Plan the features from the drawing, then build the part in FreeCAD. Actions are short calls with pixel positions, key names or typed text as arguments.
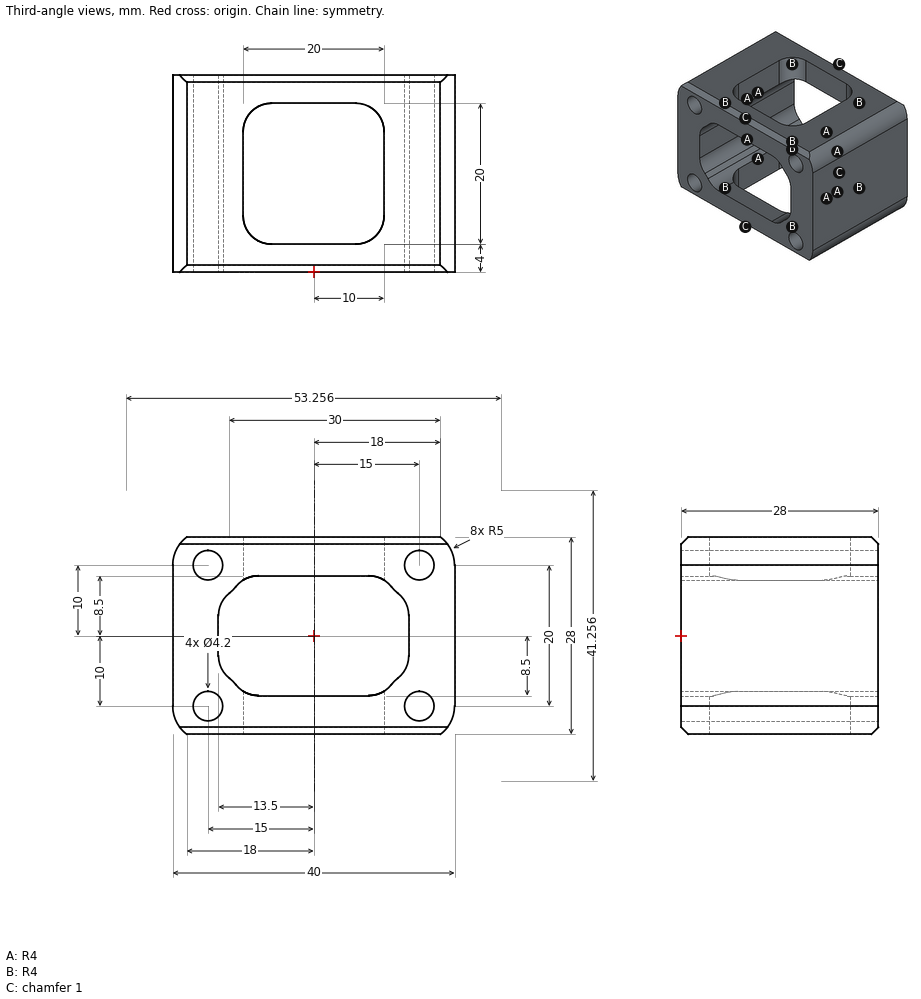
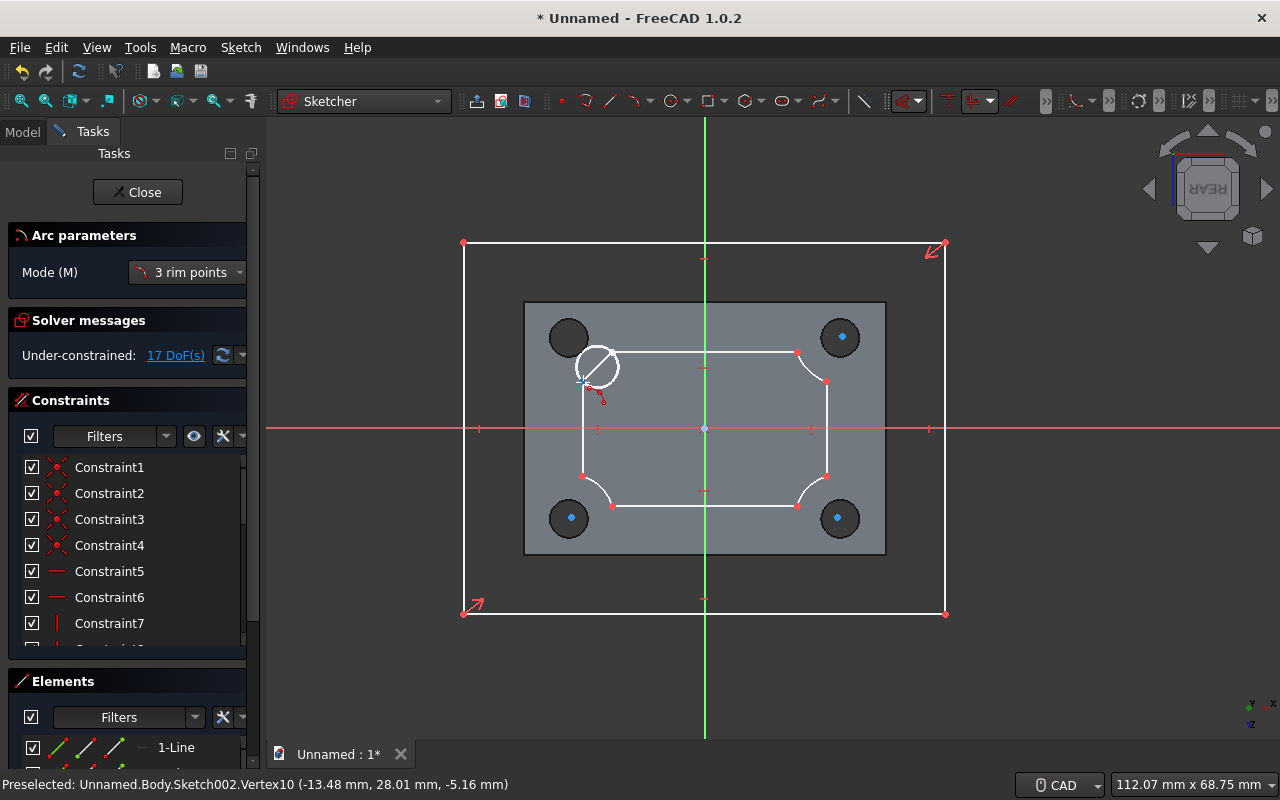
scroll(601, 370, up, 6)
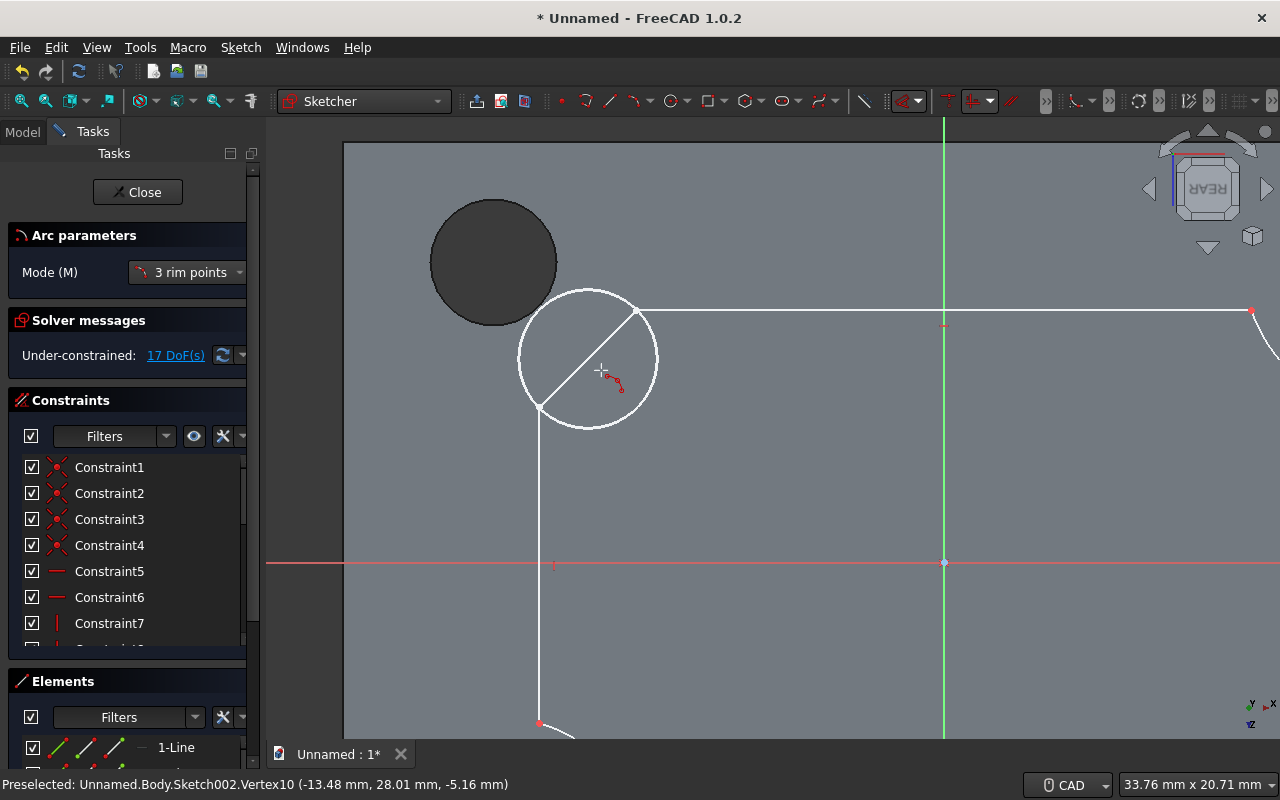
click(600, 369)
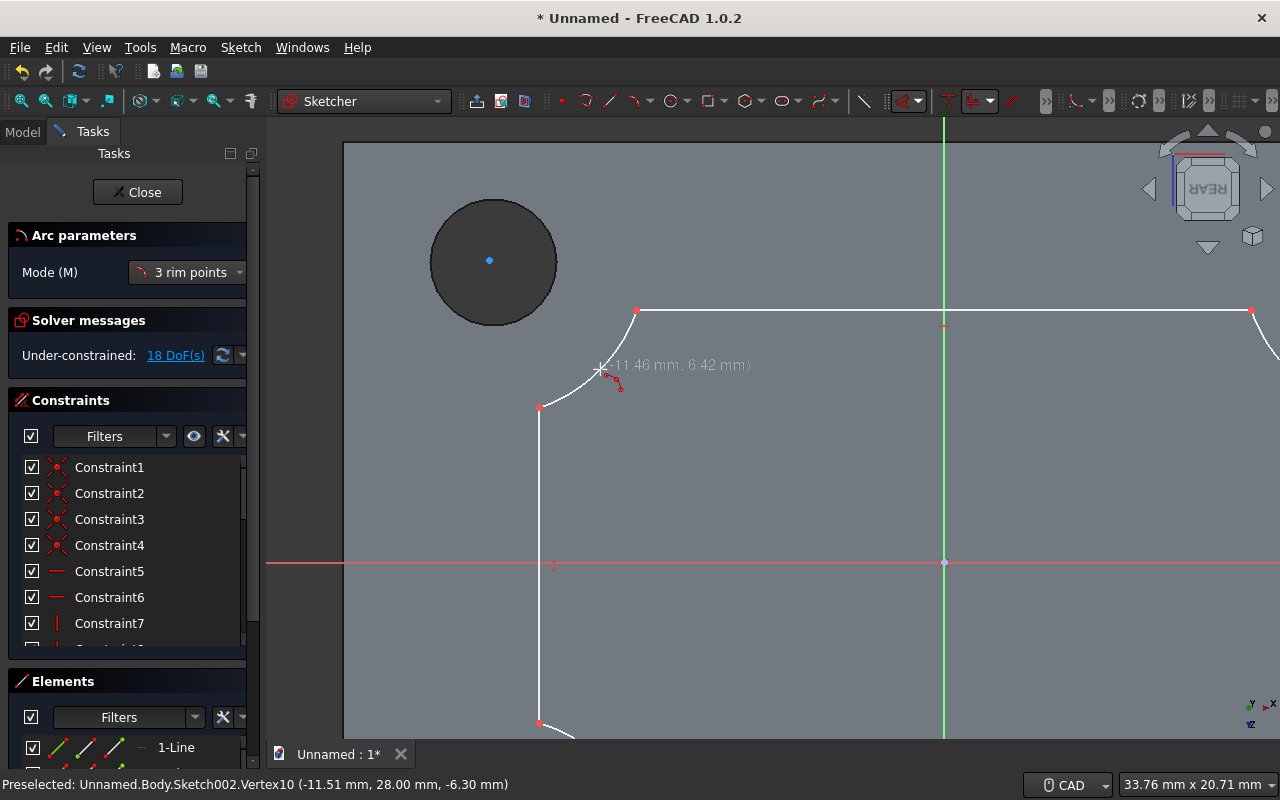
key(g)
key(l)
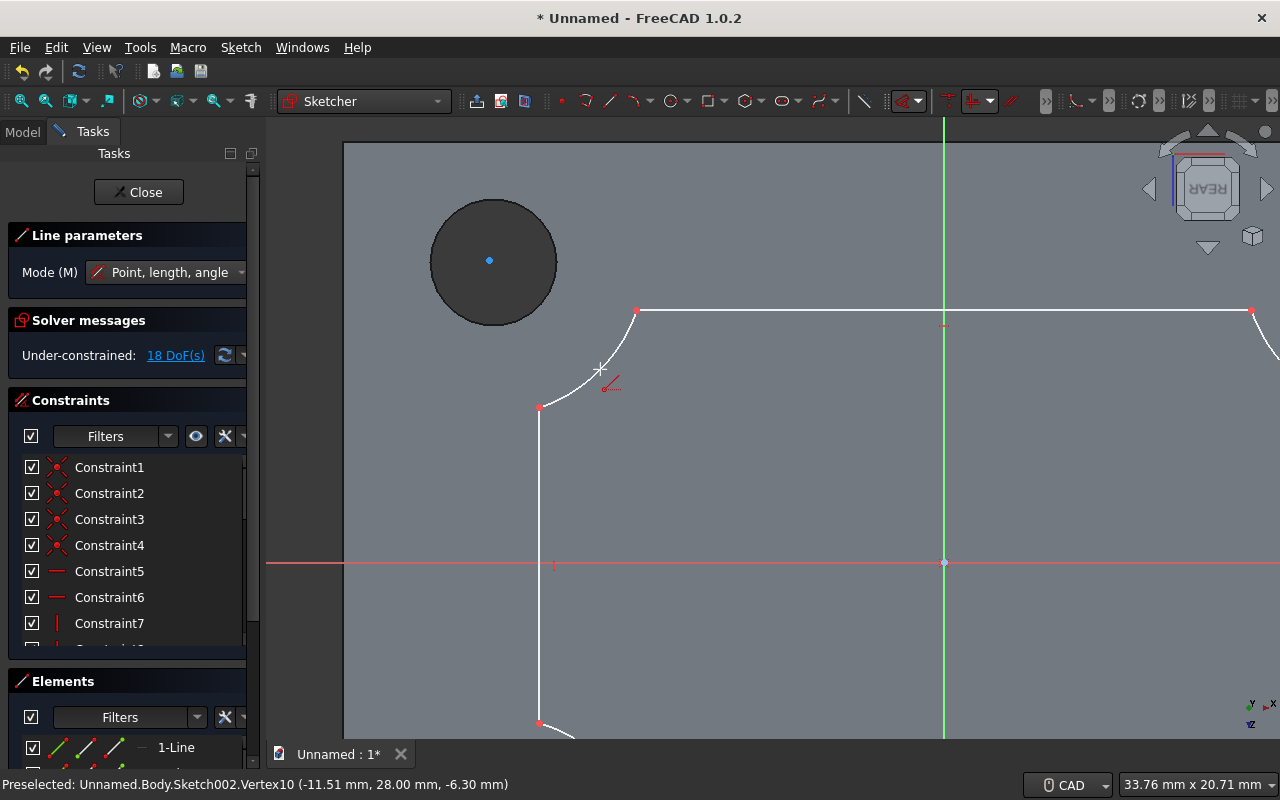
scroll(601, 370, down, 6)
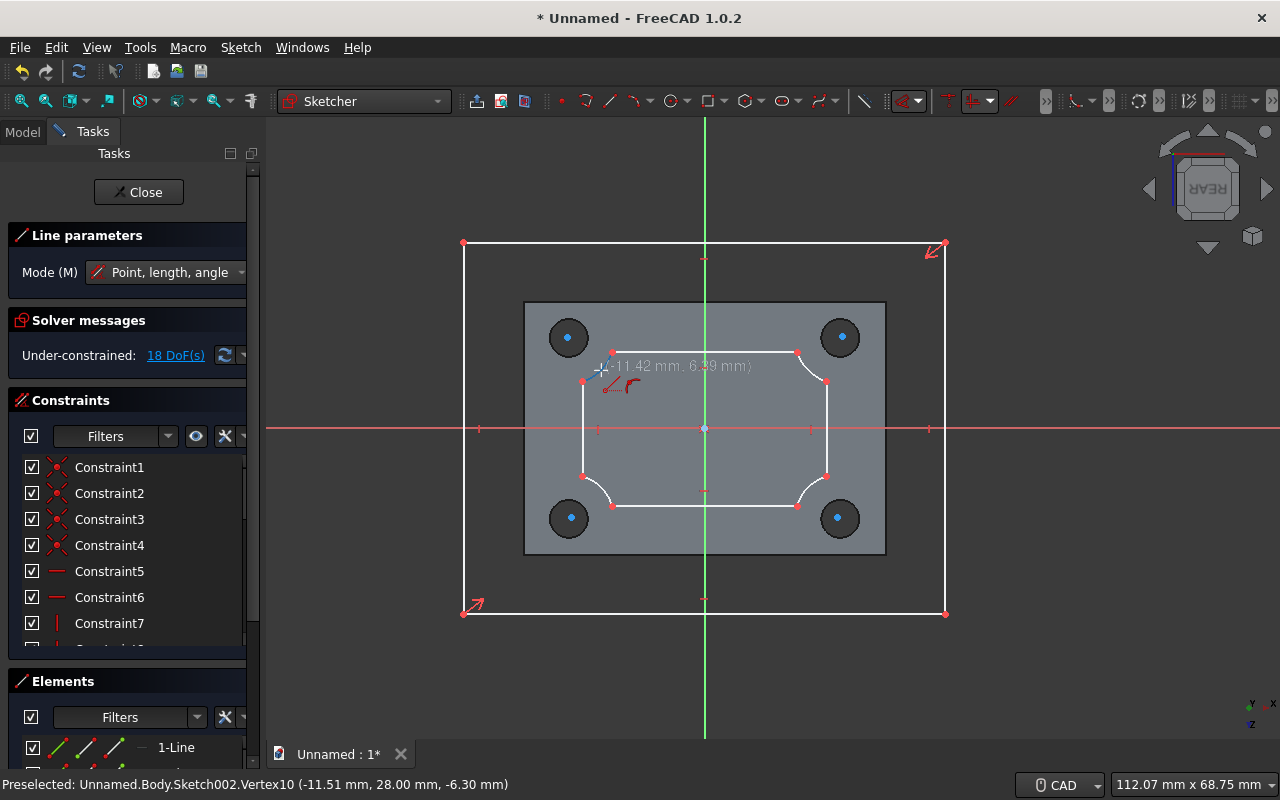
click(886, 338)
click(886, 519)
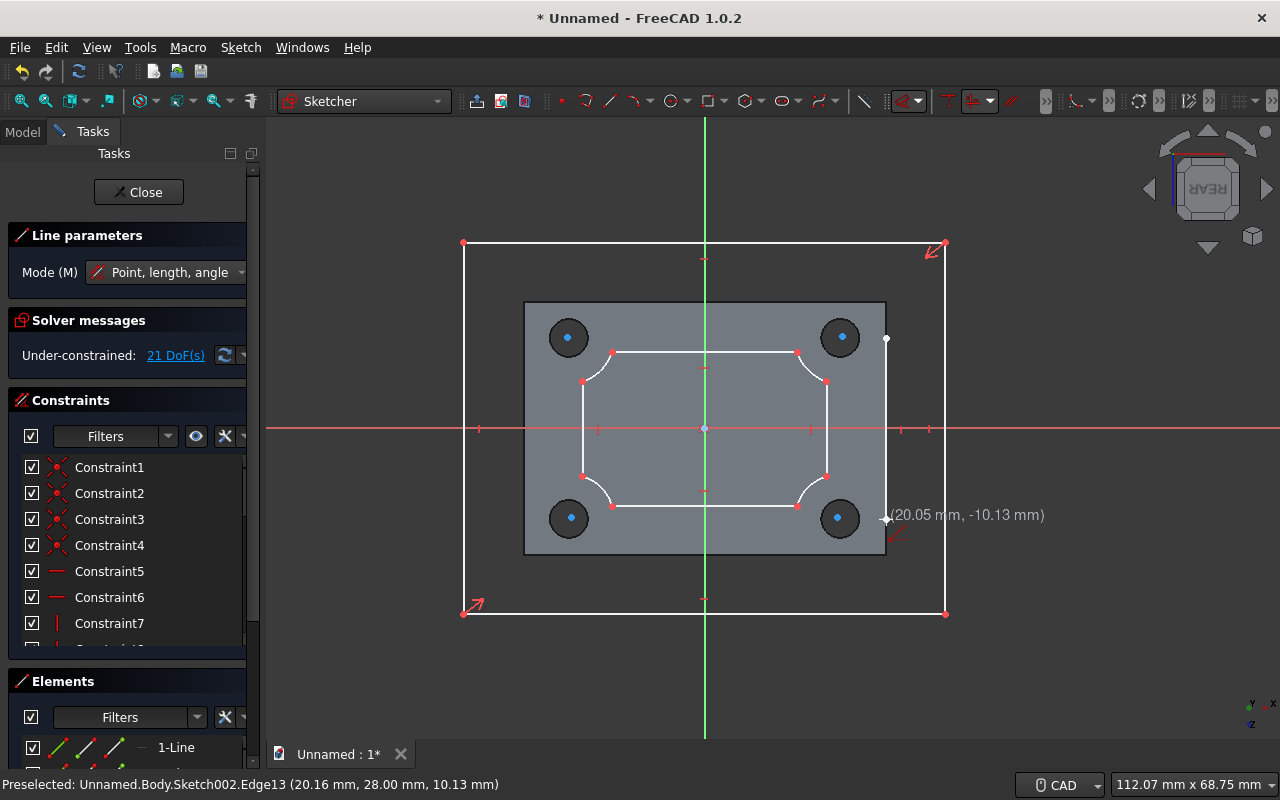
click(867, 555)
click(596, 555)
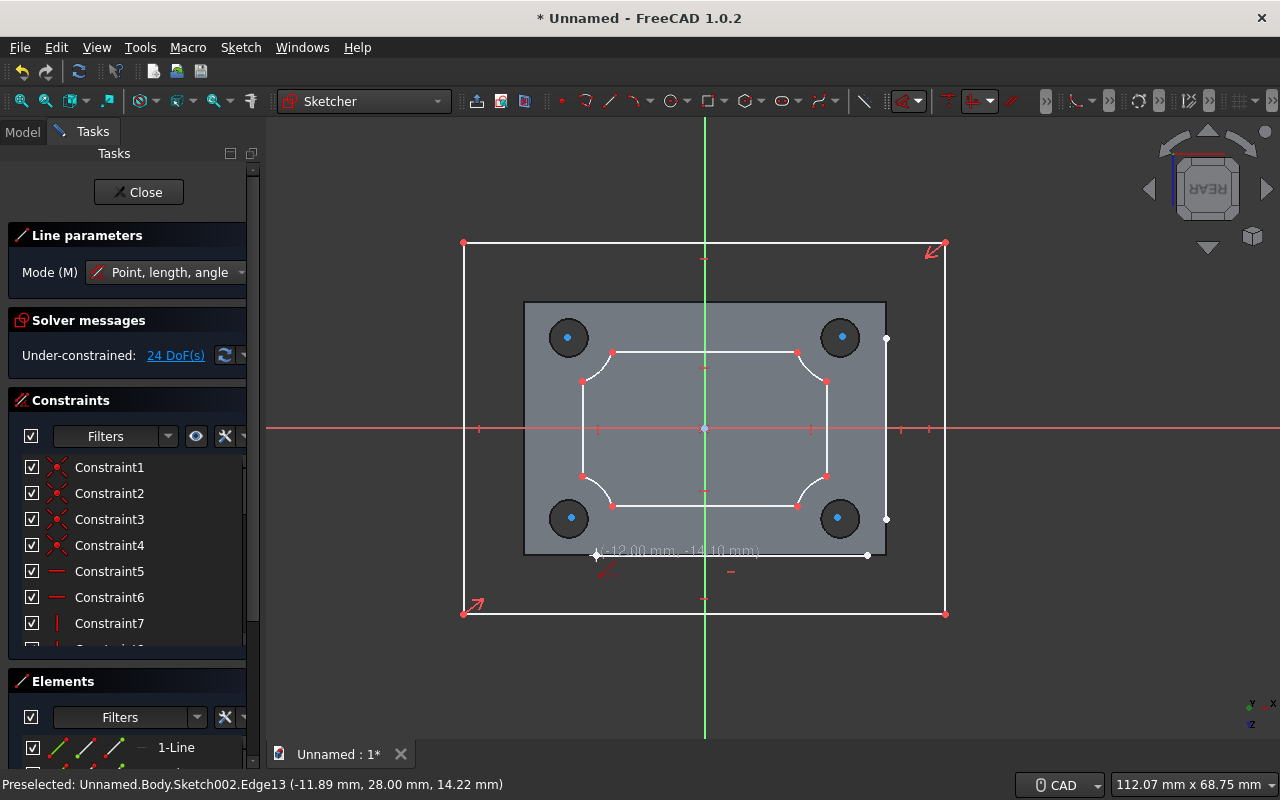
click(524, 519)
click(524, 338)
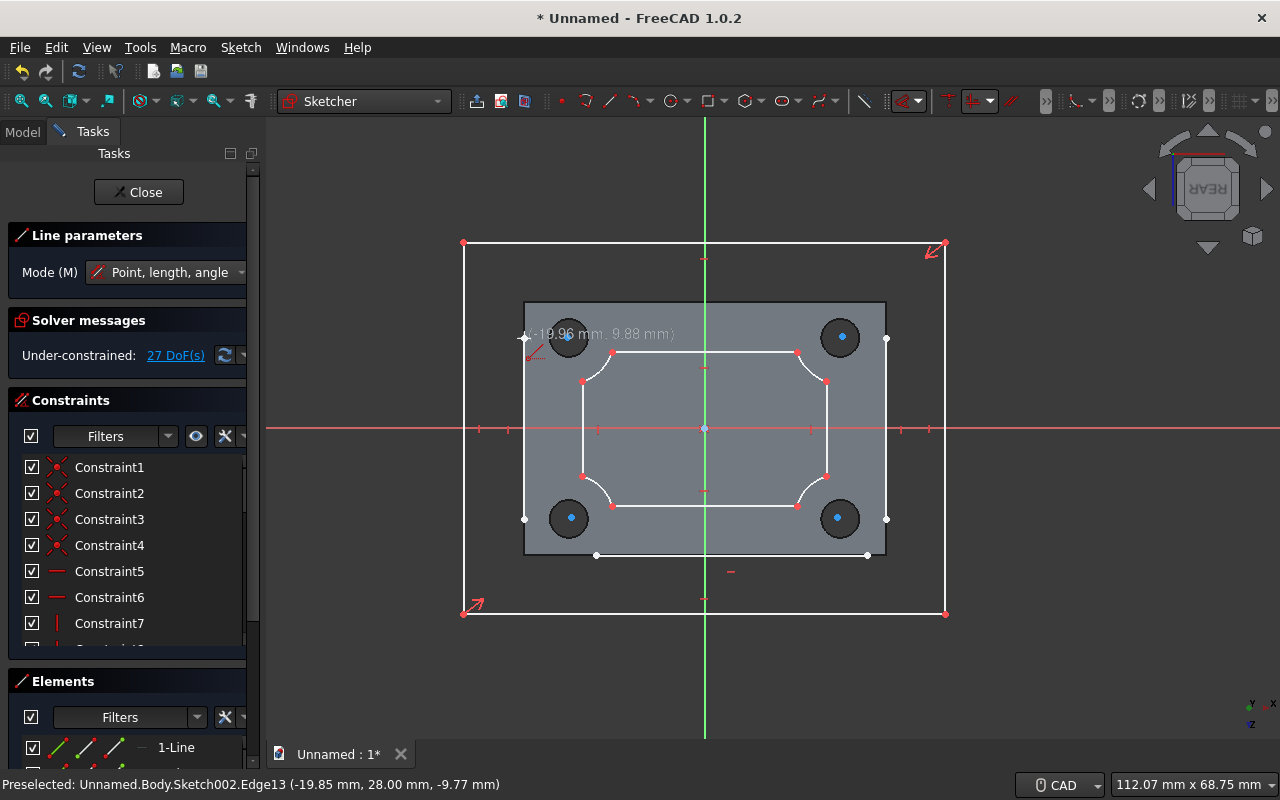
click(542, 302)
click(813, 302)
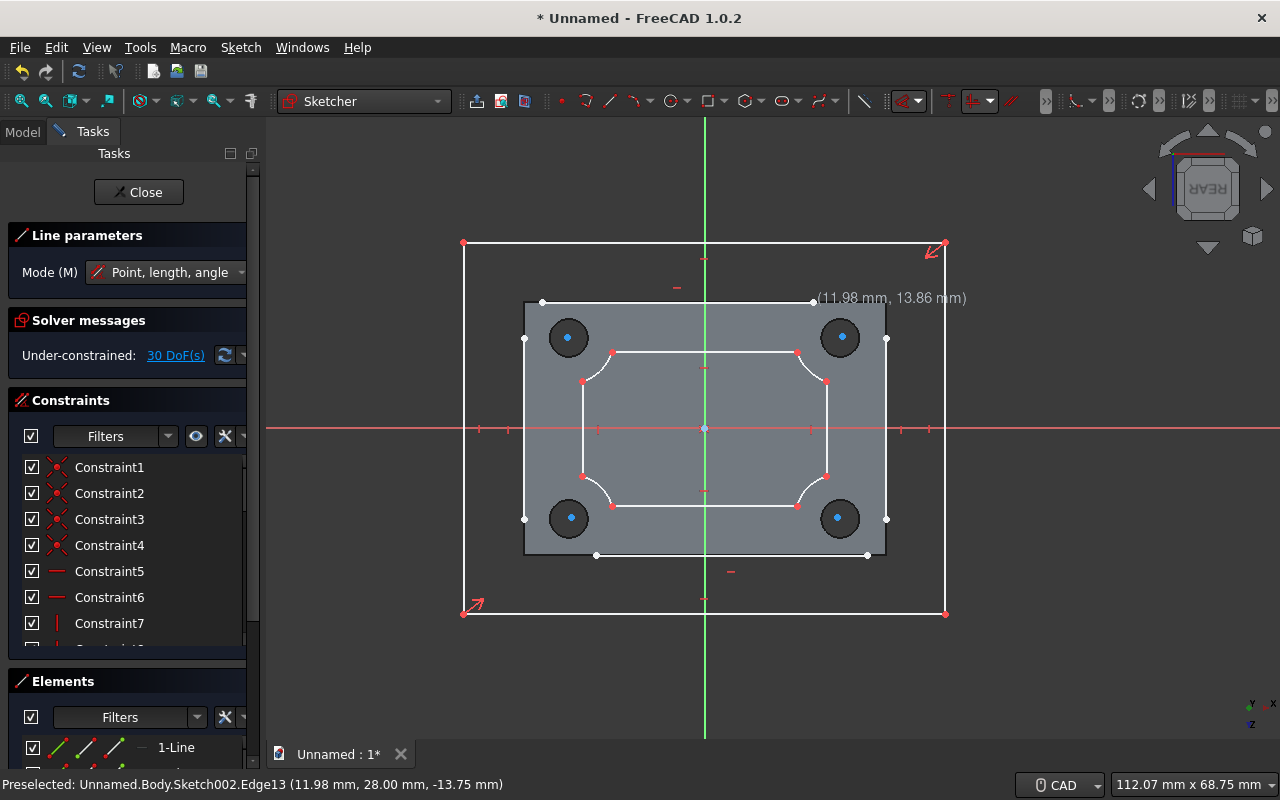
key(g)
key(3)
key(a)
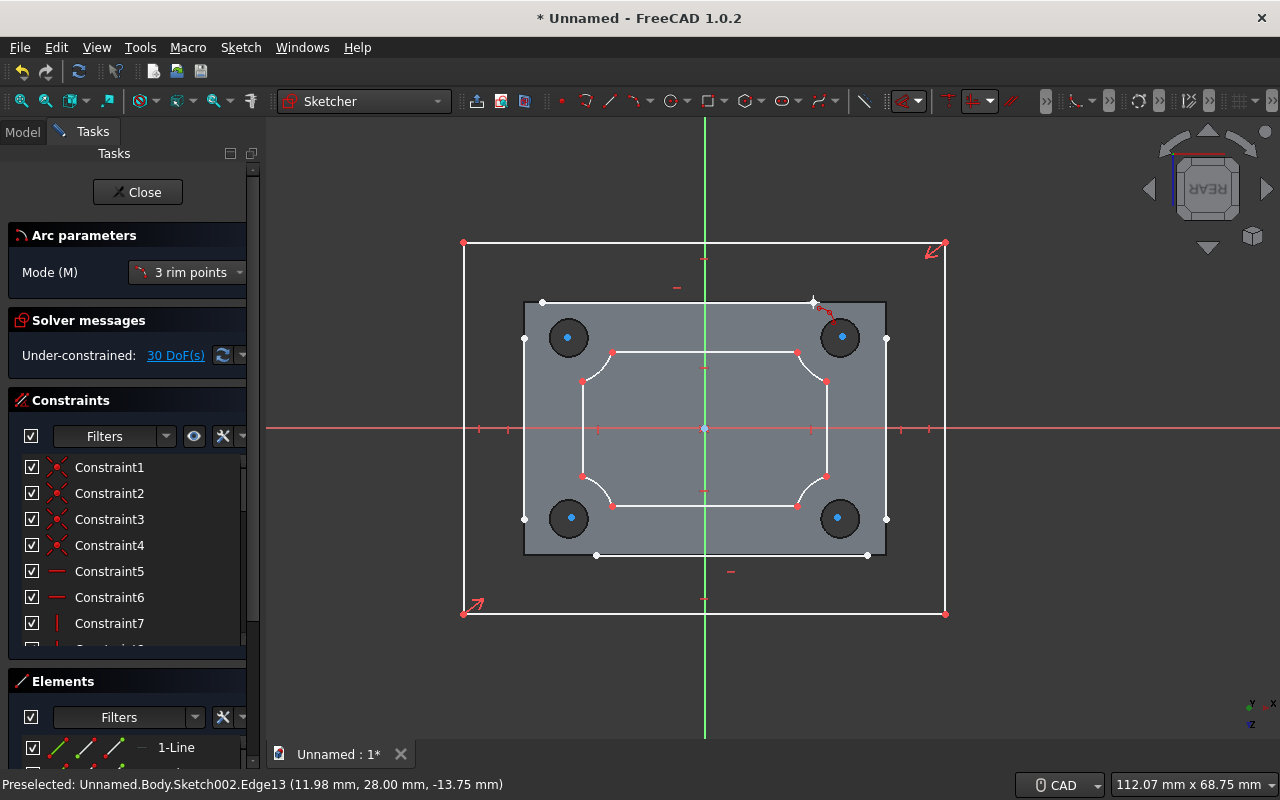
click(886, 520)
click(867, 556)